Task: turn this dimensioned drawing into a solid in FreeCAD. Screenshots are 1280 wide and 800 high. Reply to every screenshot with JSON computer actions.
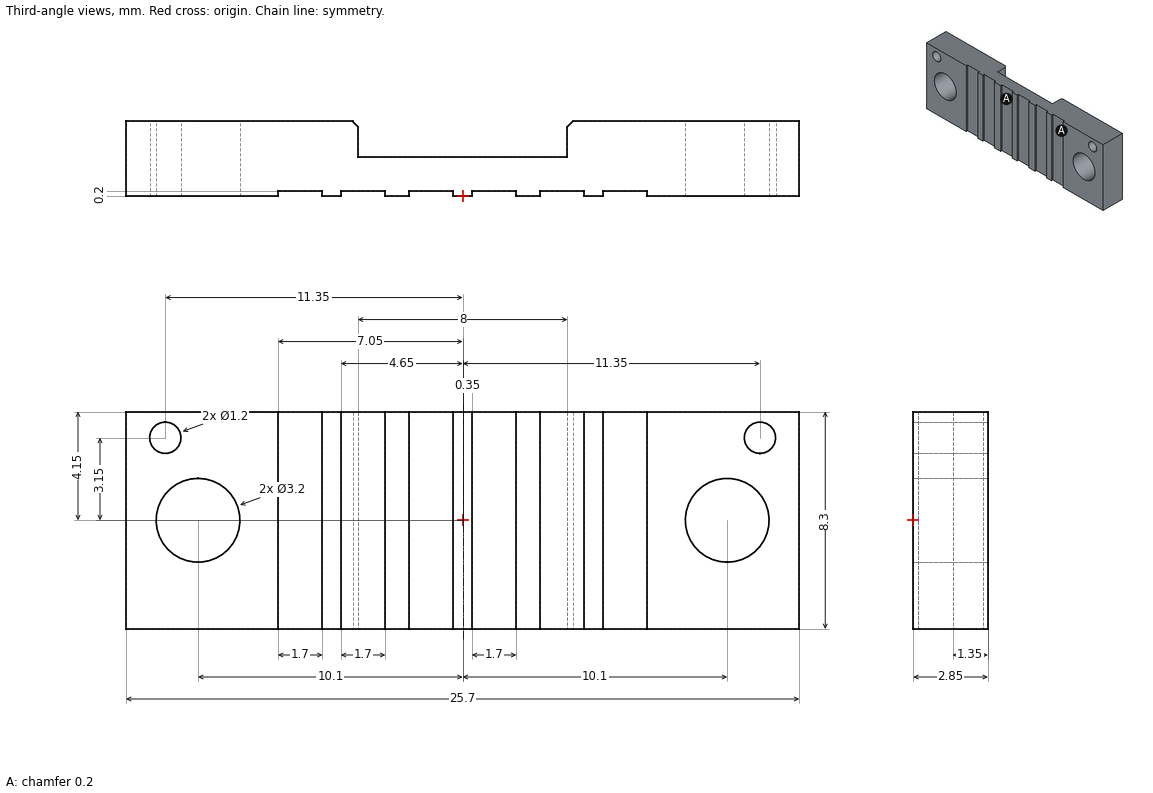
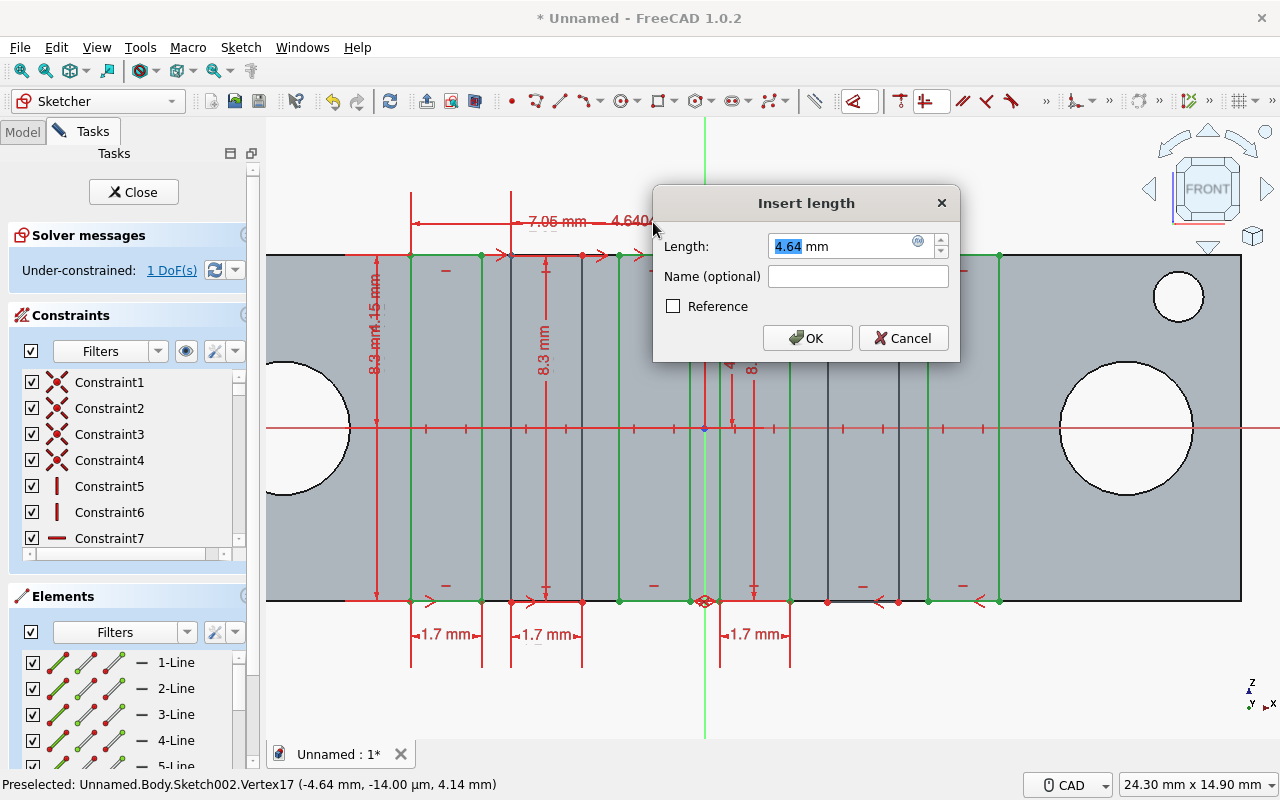
{"action": "type", "text": "4.65"}
{"action": "key", "text": "Return"}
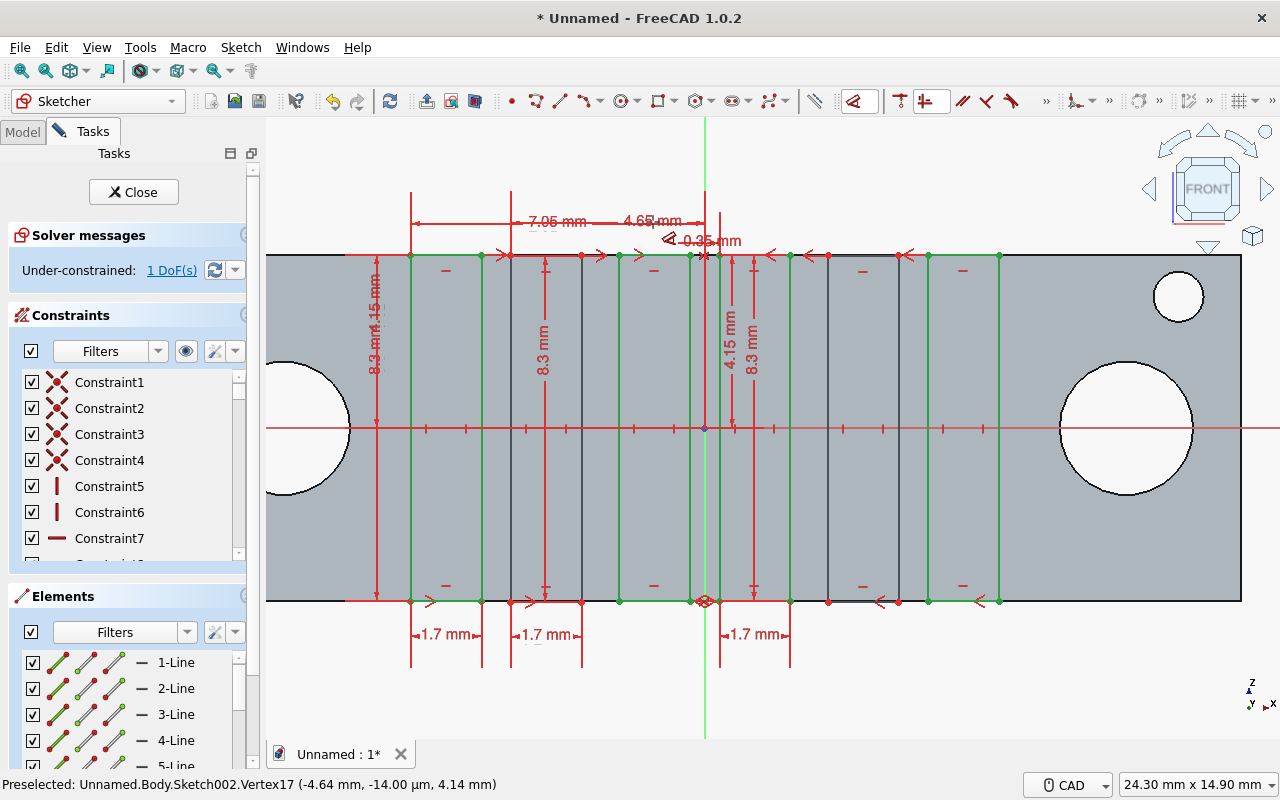
{"action": "left_click", "coordinate": [511, 256]}
{"action": "left_click", "coordinate": [739, 302]}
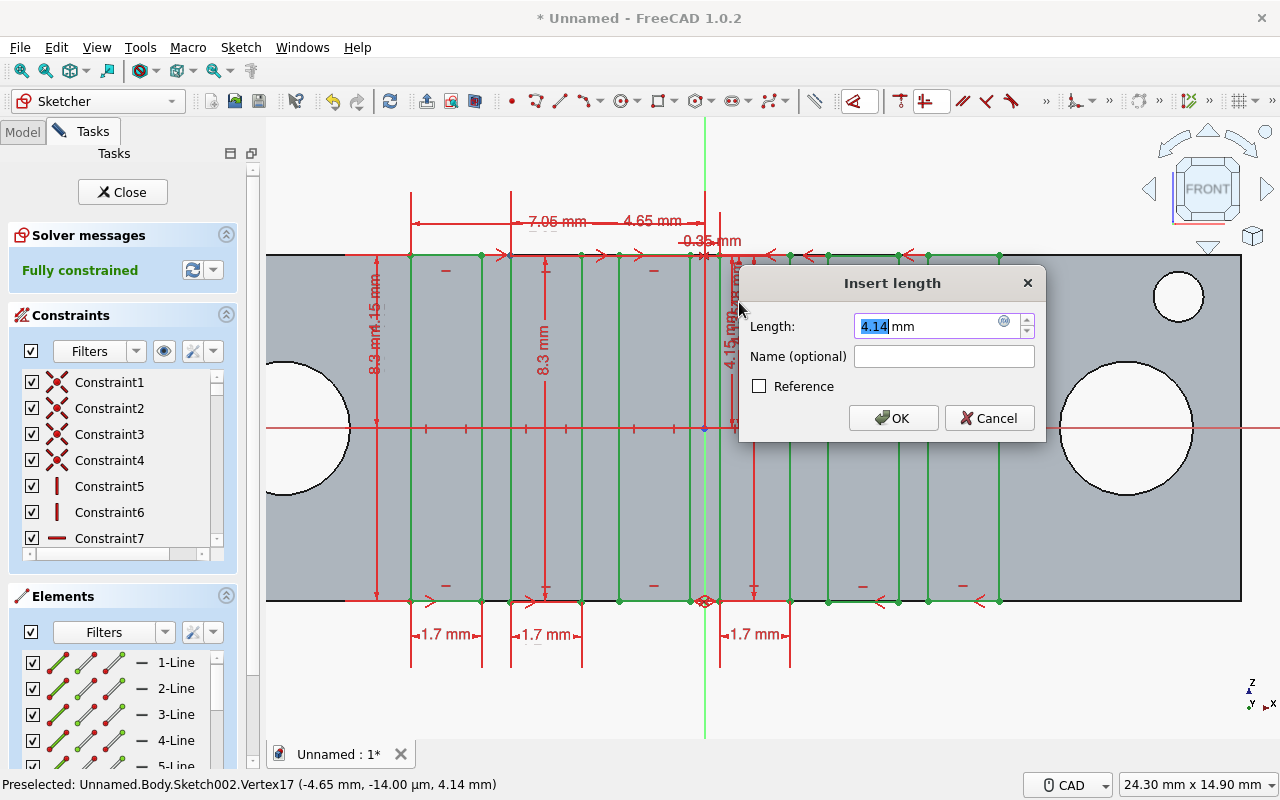
{"action": "type", "text": "4.15"}
{"action": "key", "text": "Return"}
{"action": "key", "text": "Escape"}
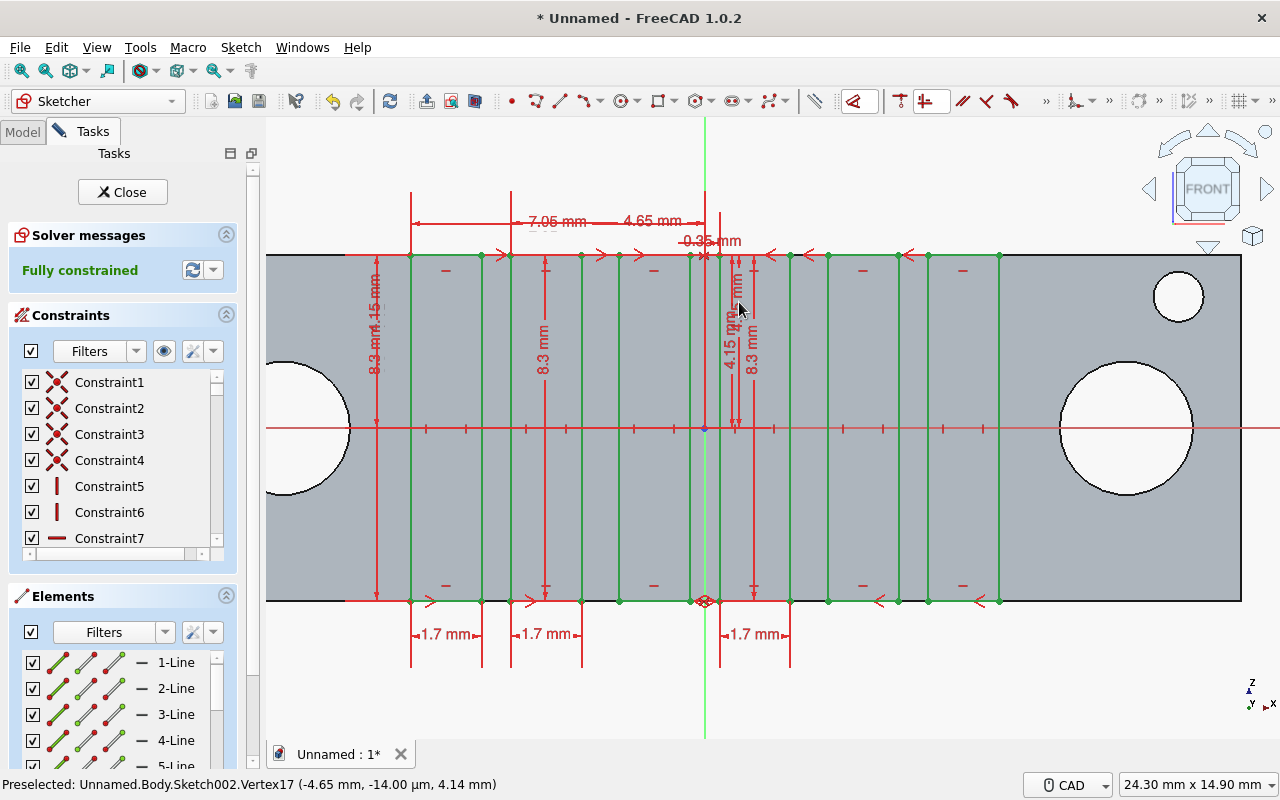
{"action": "left_click", "coordinate": [123, 192]}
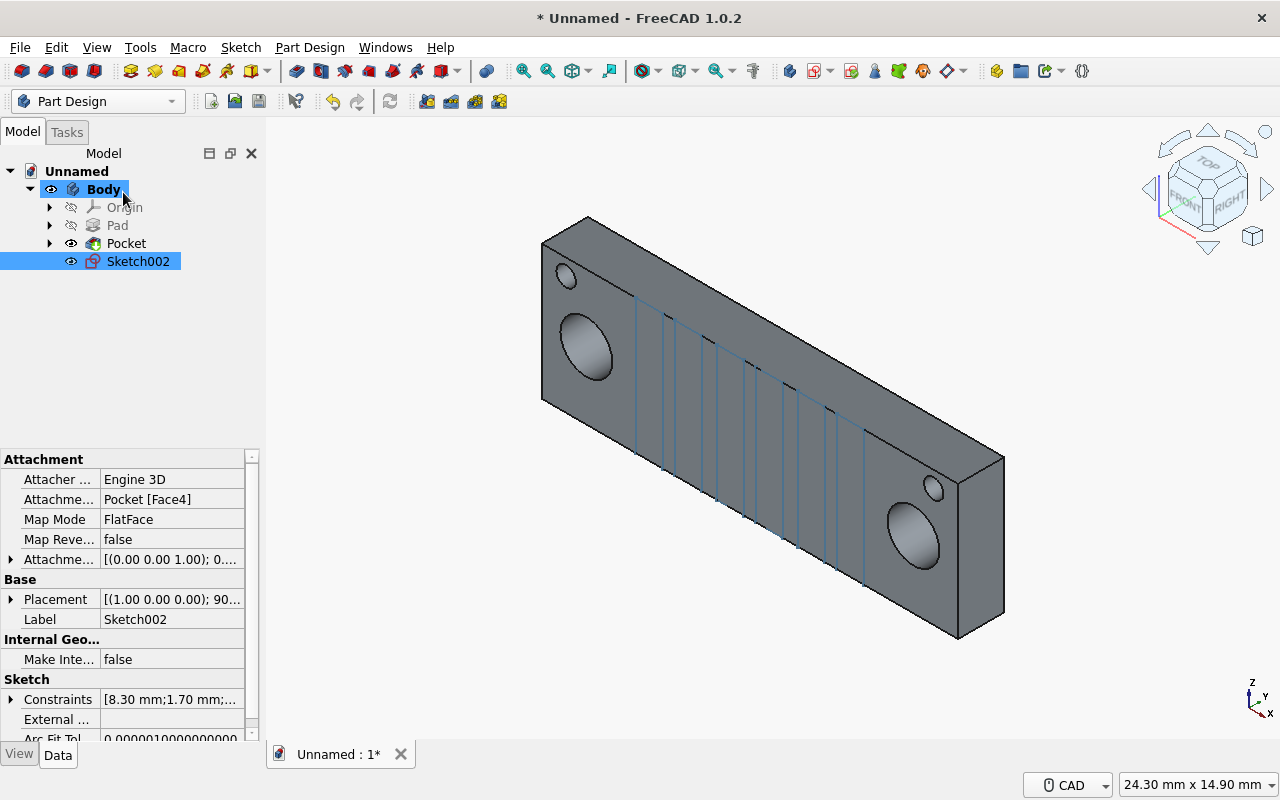
{"action": "left_click", "coordinate": [298, 72]}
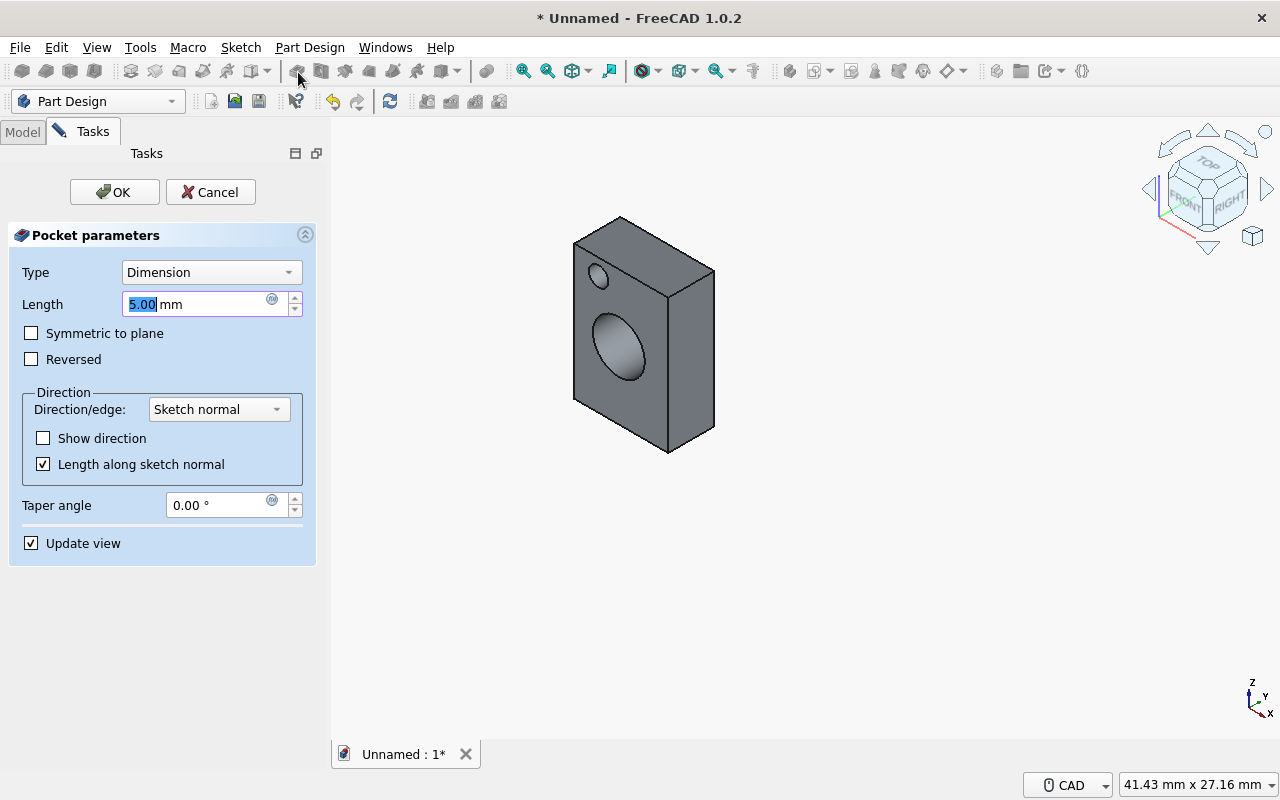
{"action": "type", "text": "0.2"}
{"action": "key", "text": "Tab"}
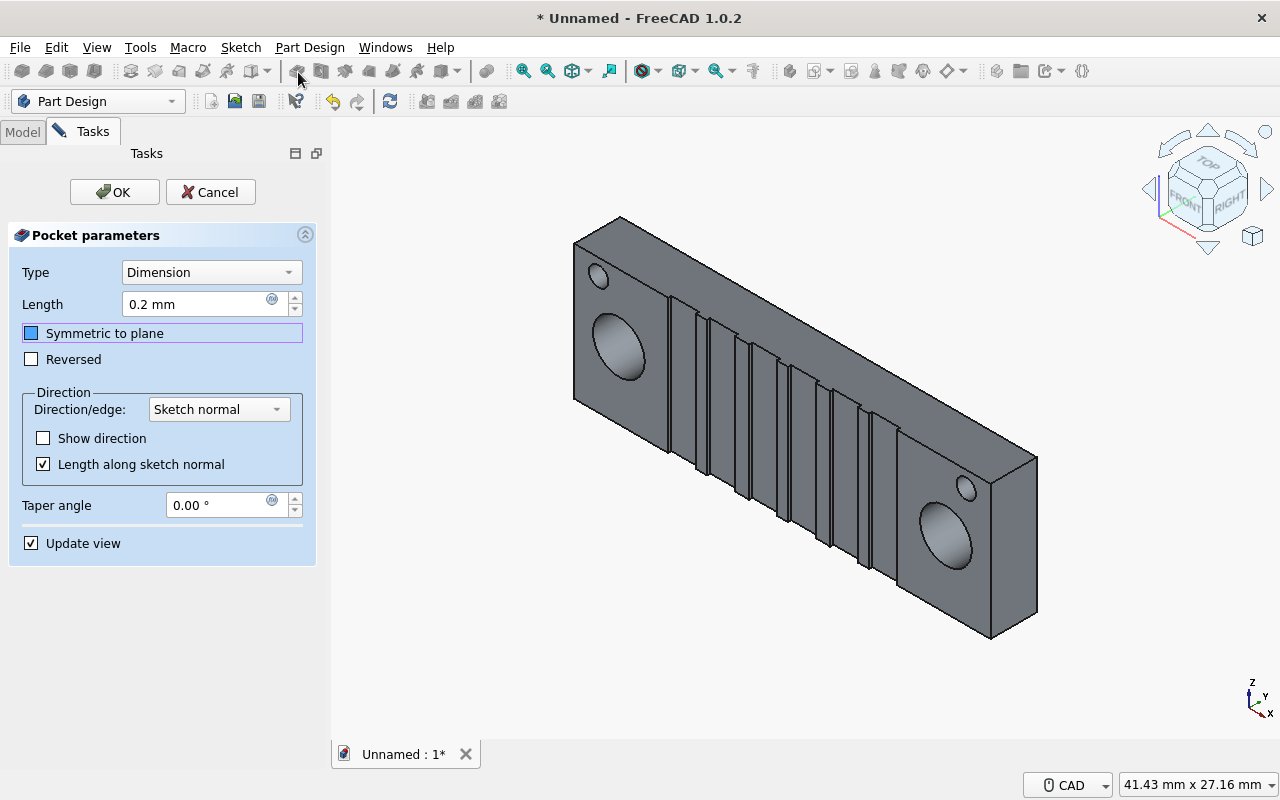
{"action": "left_click", "coordinate": [115, 192]}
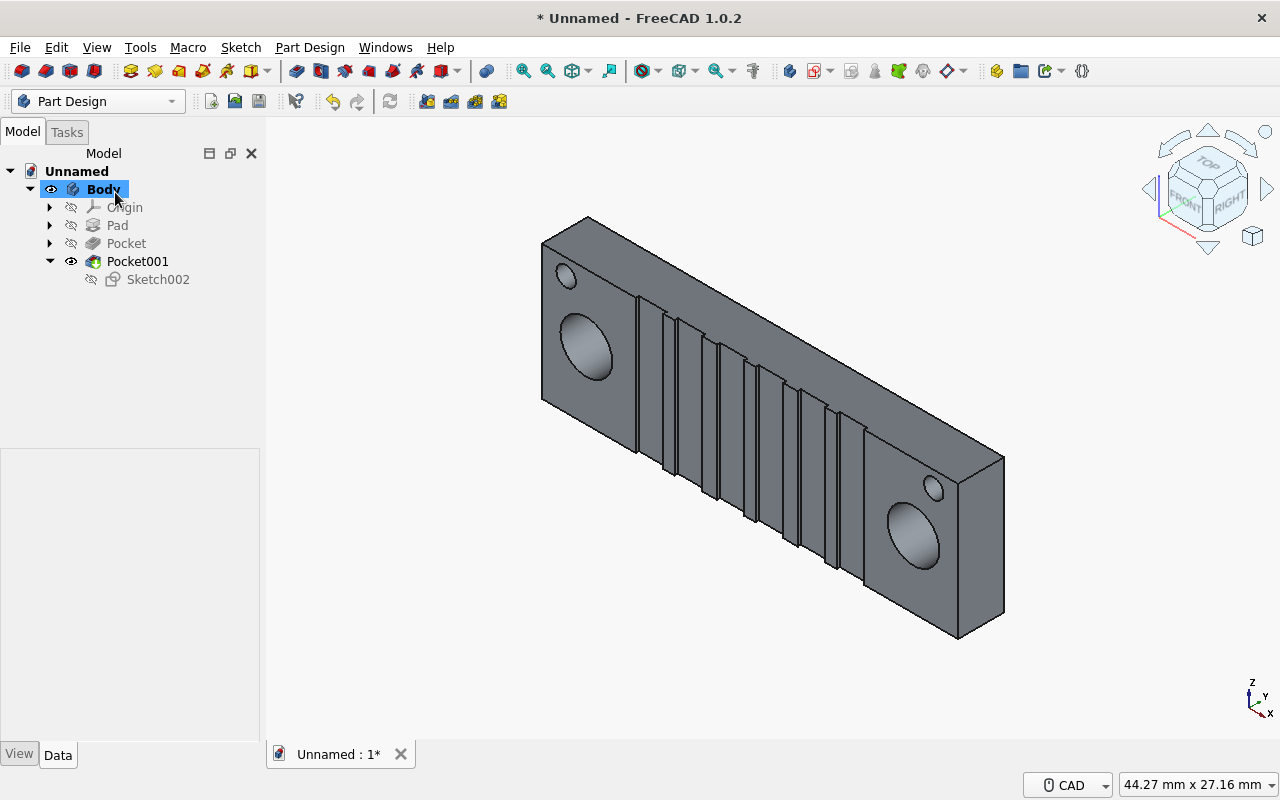
{"action": "key", "text": "4"}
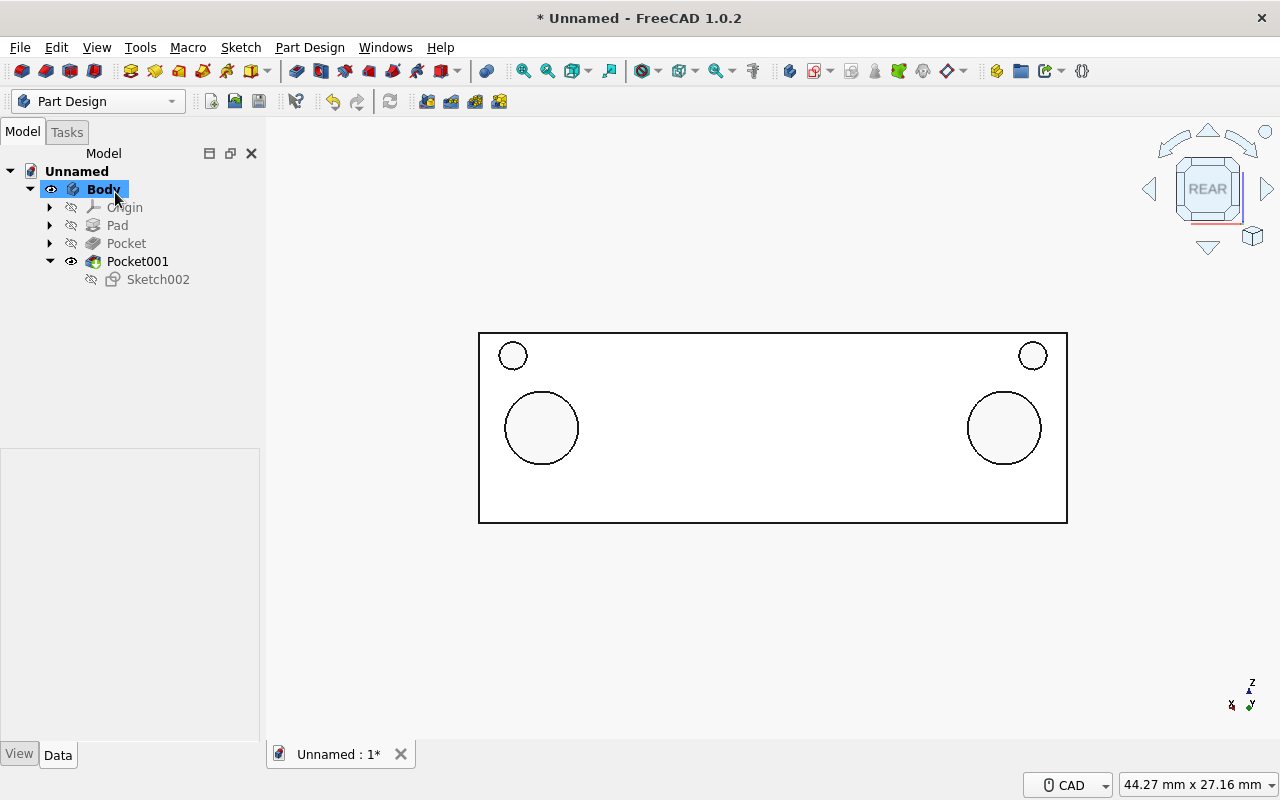
{"action": "left_click", "coordinate": [689, 427]}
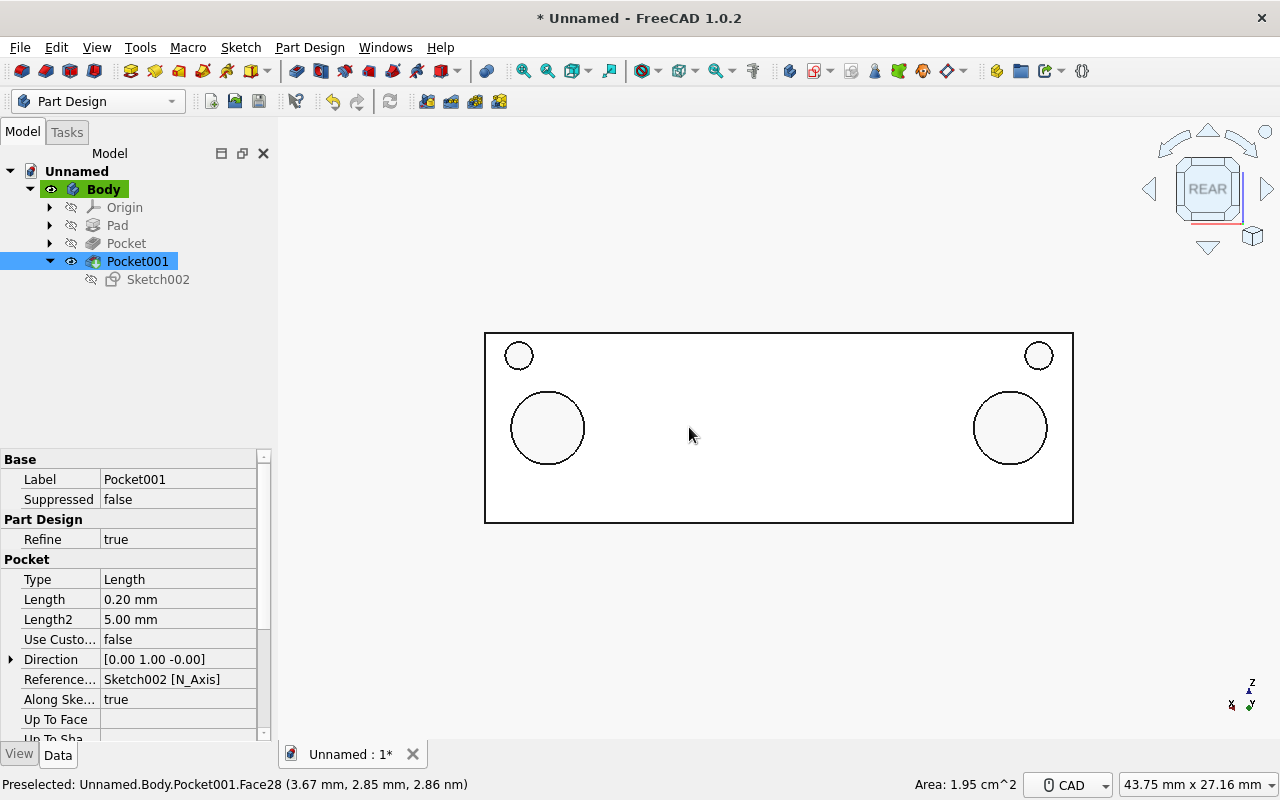
{"action": "left_click", "coordinate": [814, 72]}